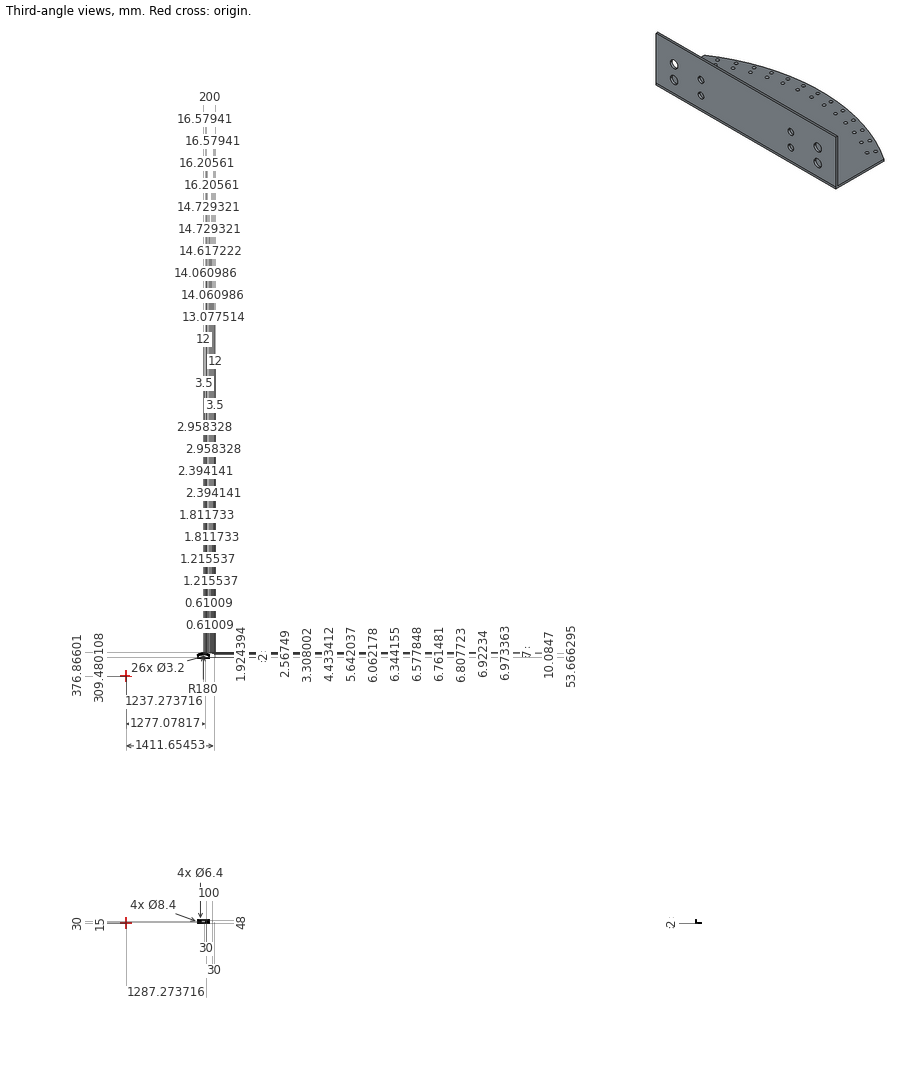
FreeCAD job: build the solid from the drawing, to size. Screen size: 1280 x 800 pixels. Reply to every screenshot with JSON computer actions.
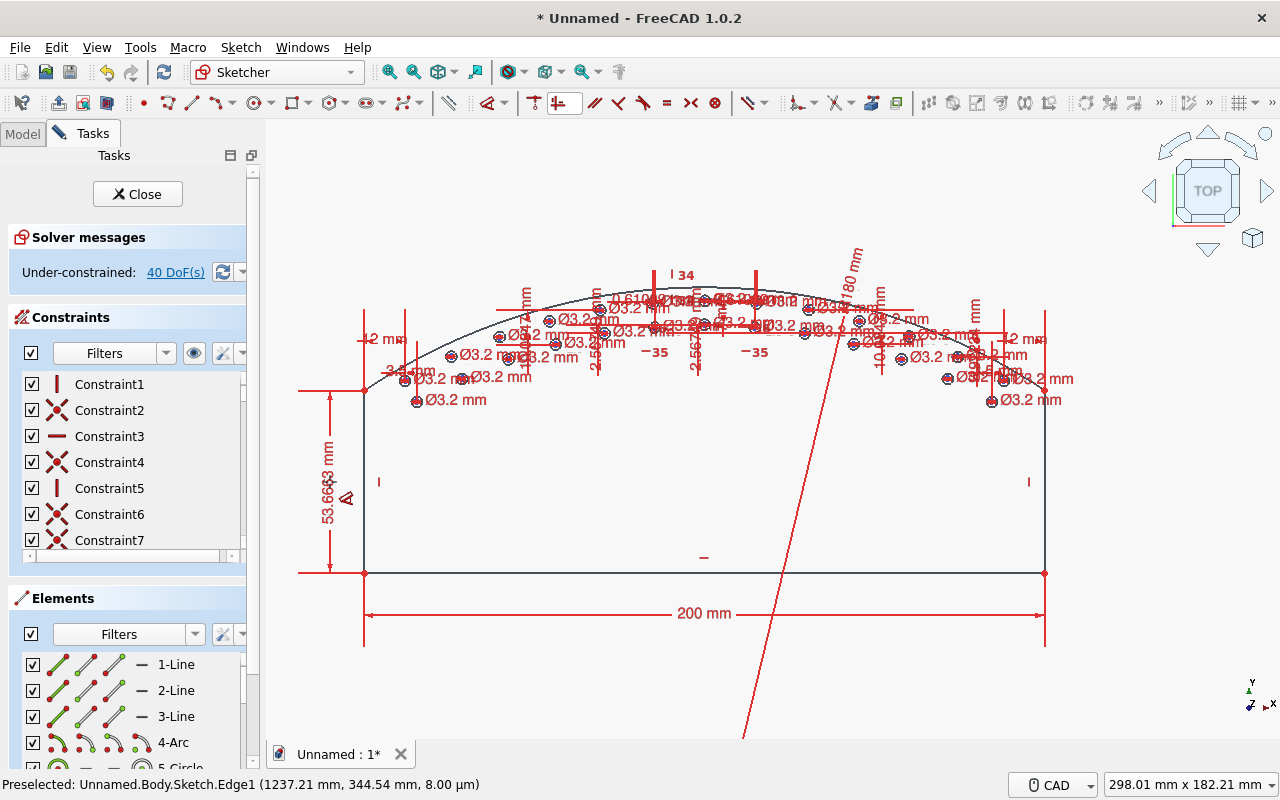
{"action": "left_click", "coordinate": [1045, 518]}
{"action": "left_click", "coordinate": [1079, 482]}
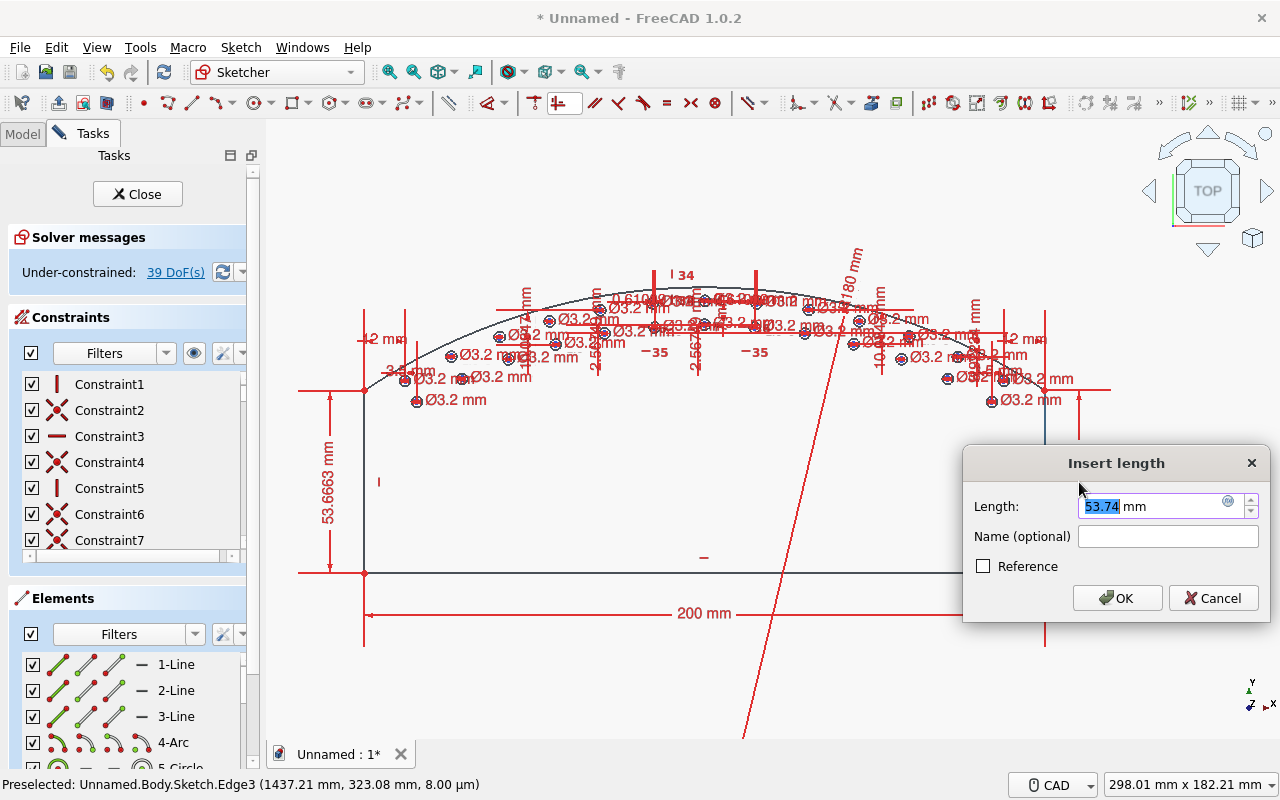
{"action": "type", "text": "53.666295"}
{"action": "key", "text": "Return"}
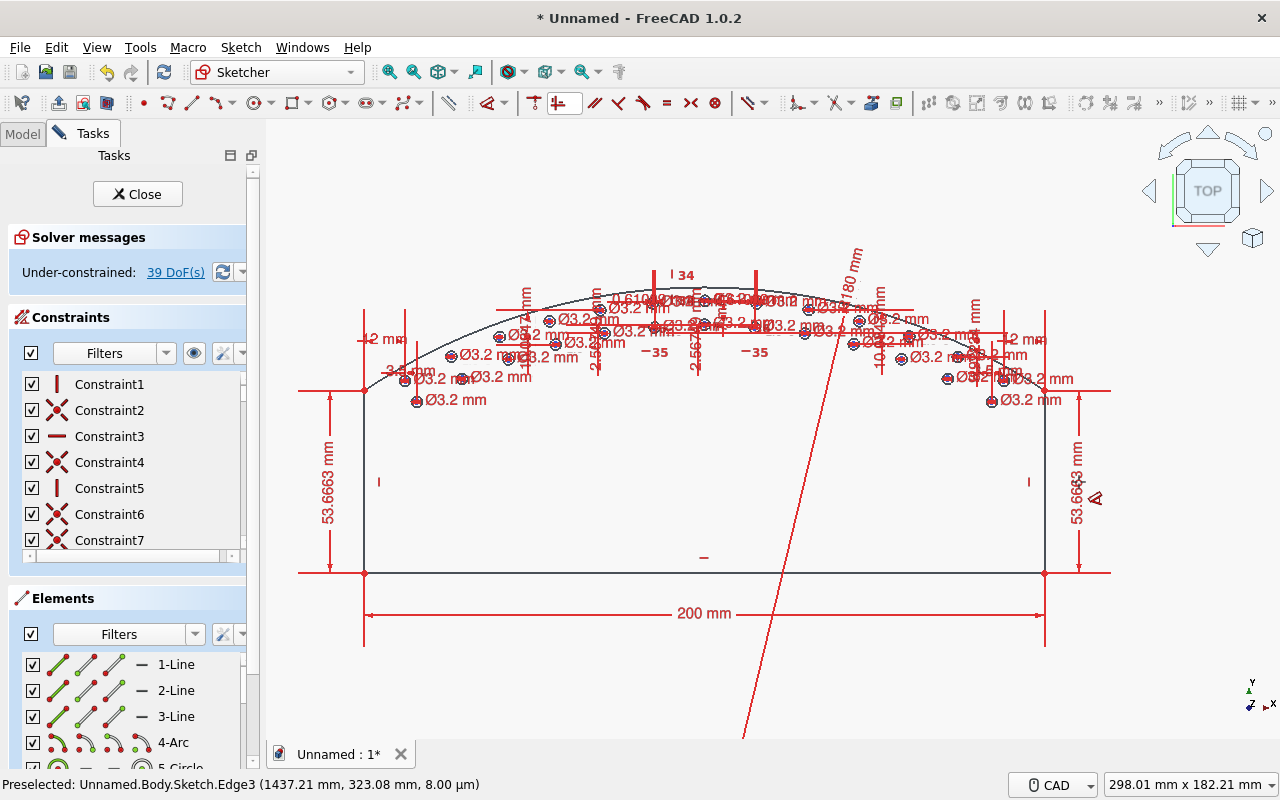
{"action": "left_click", "coordinate": [909, 337]}
{"action": "left_click", "coordinate": [943, 524]}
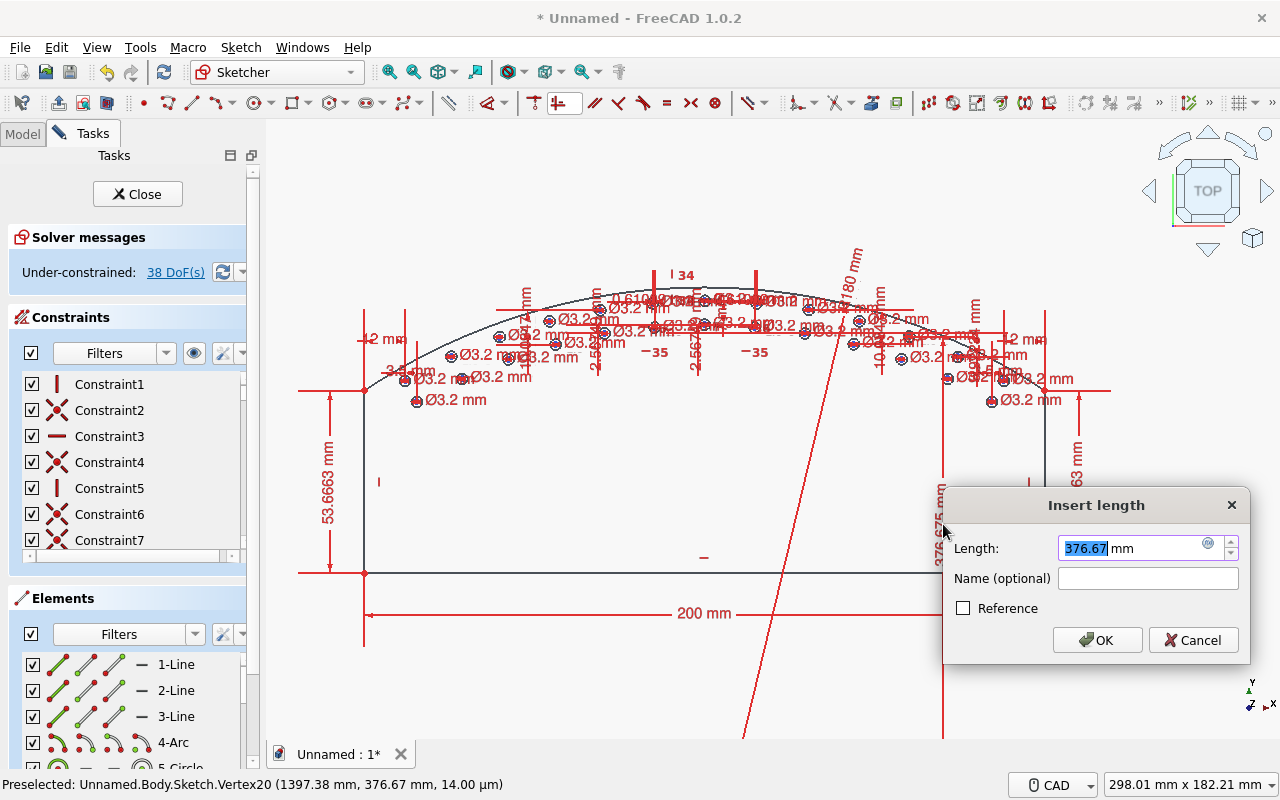
{"action": "type", "text": "376.86601"}
{"action": "key", "text": "Return"}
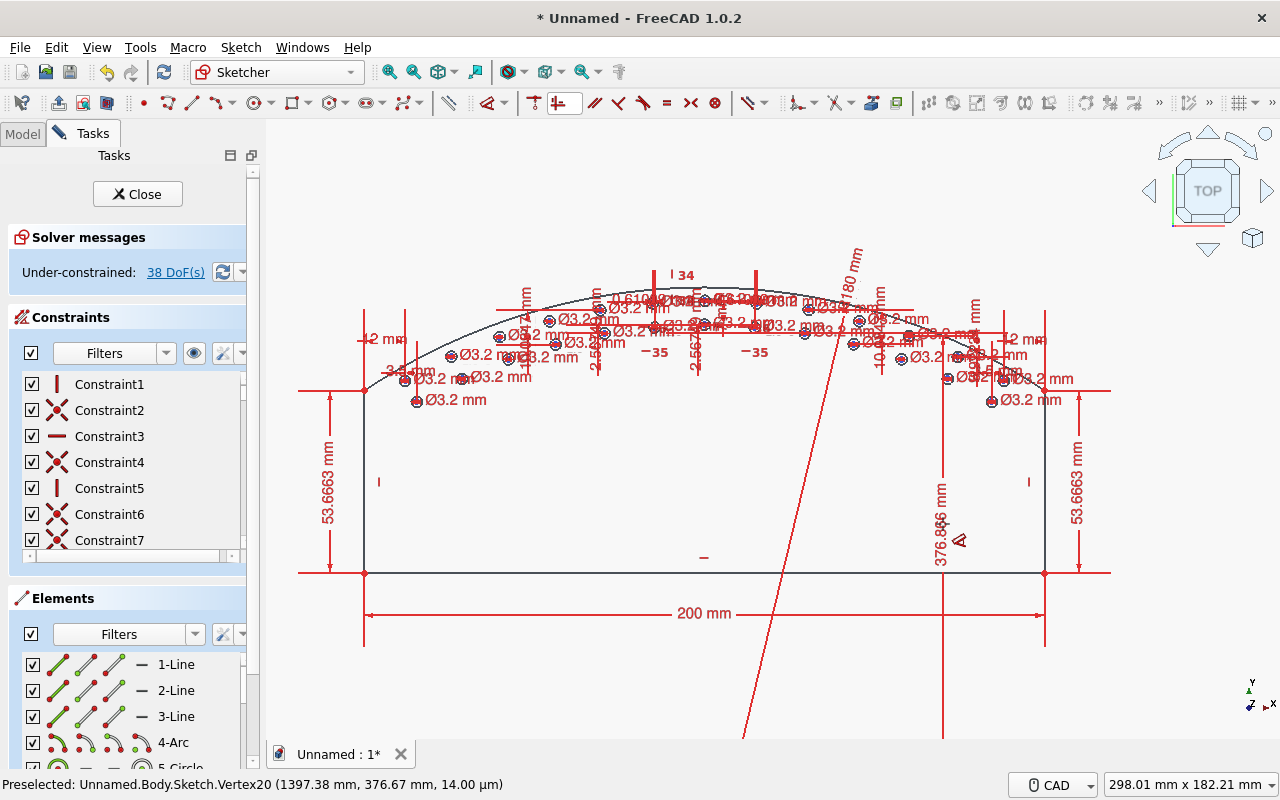
{"action": "left_click", "coordinate": [500, 337]}
{"action": "left_click", "coordinate": [534, 524]}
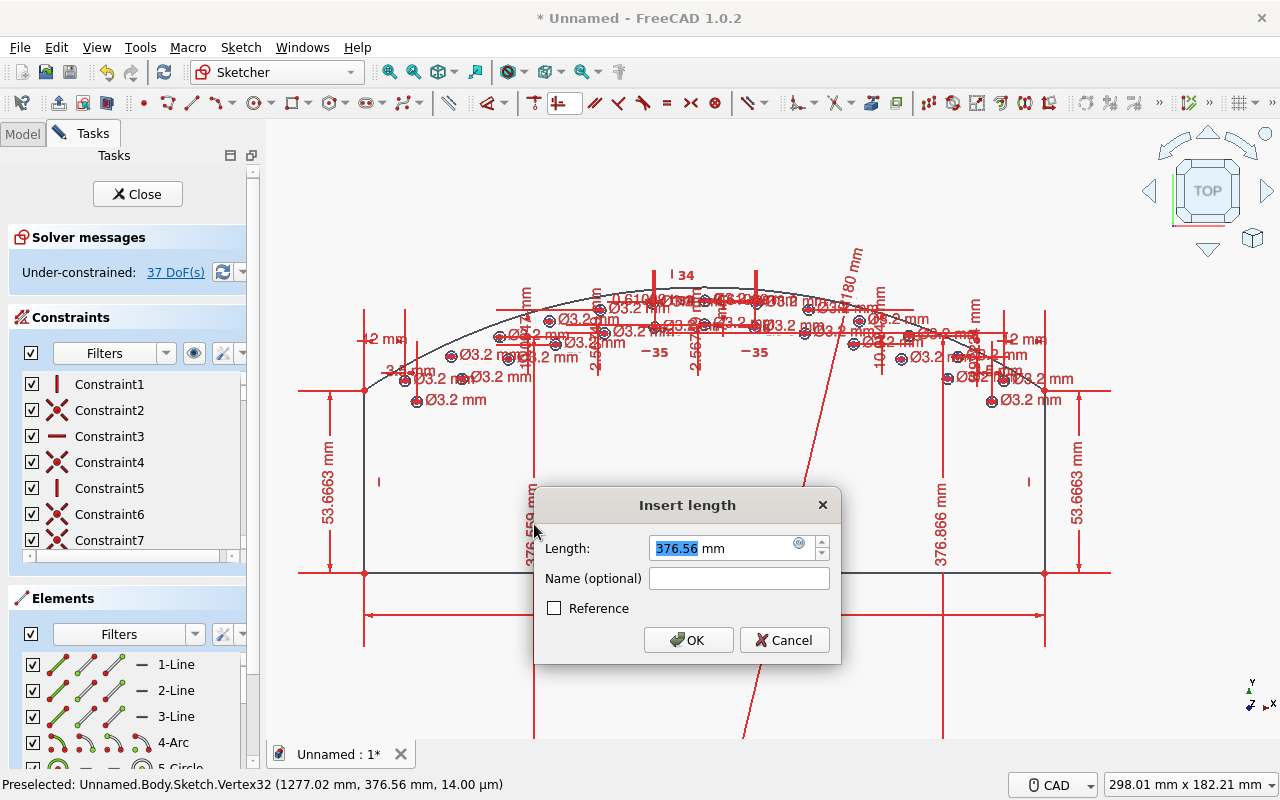
{"action": "type", "text": "376.86601"}
{"action": "key", "text": "Return"}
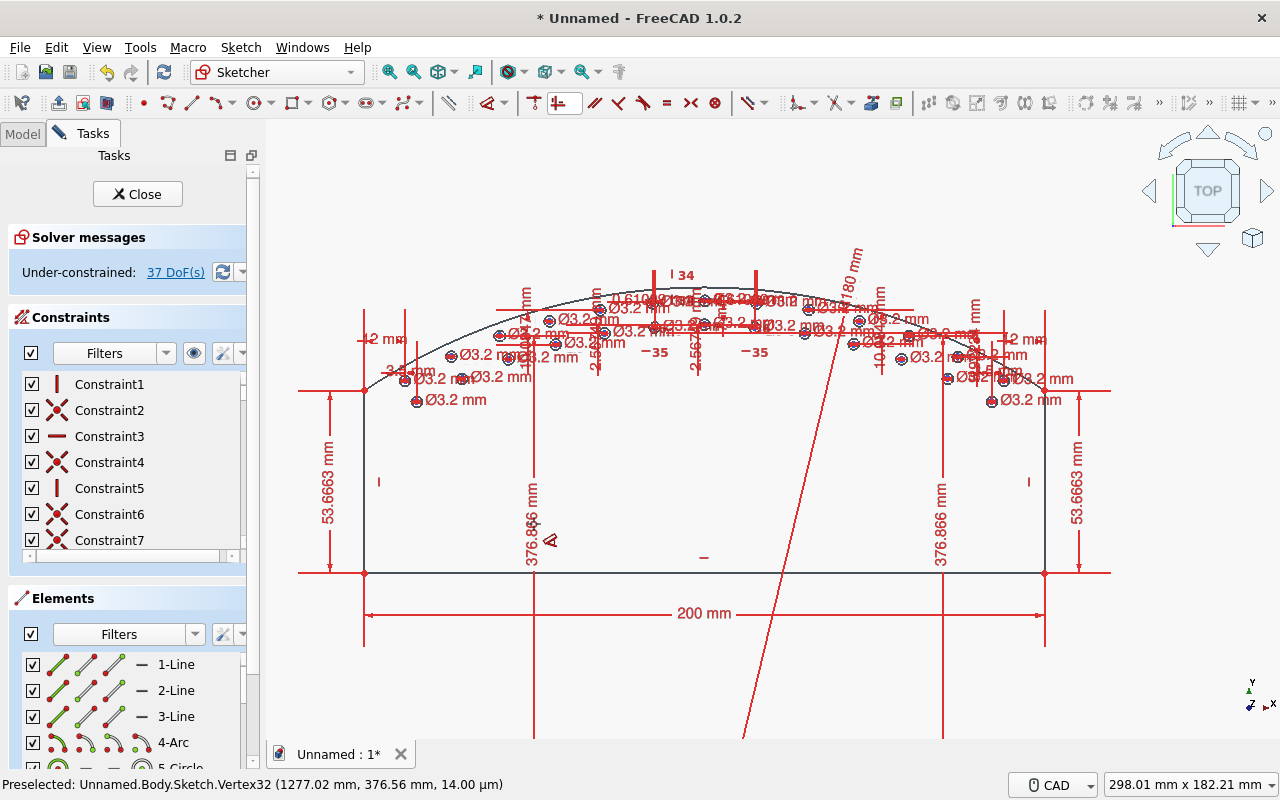
{"action": "scroll", "coordinate": [1045, 391], "scroll_direction": "up", "scroll_amount": 7}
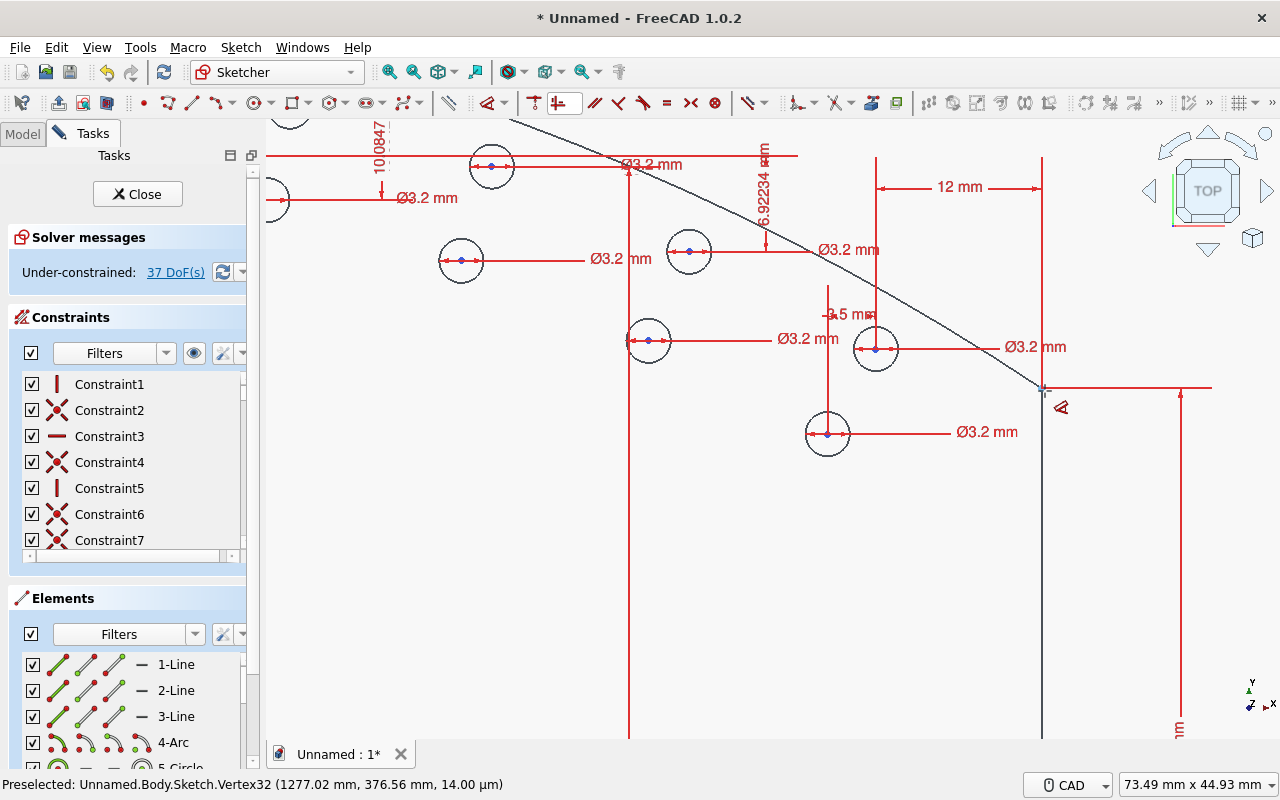
{"action": "left_click", "coordinate": [1042, 388]}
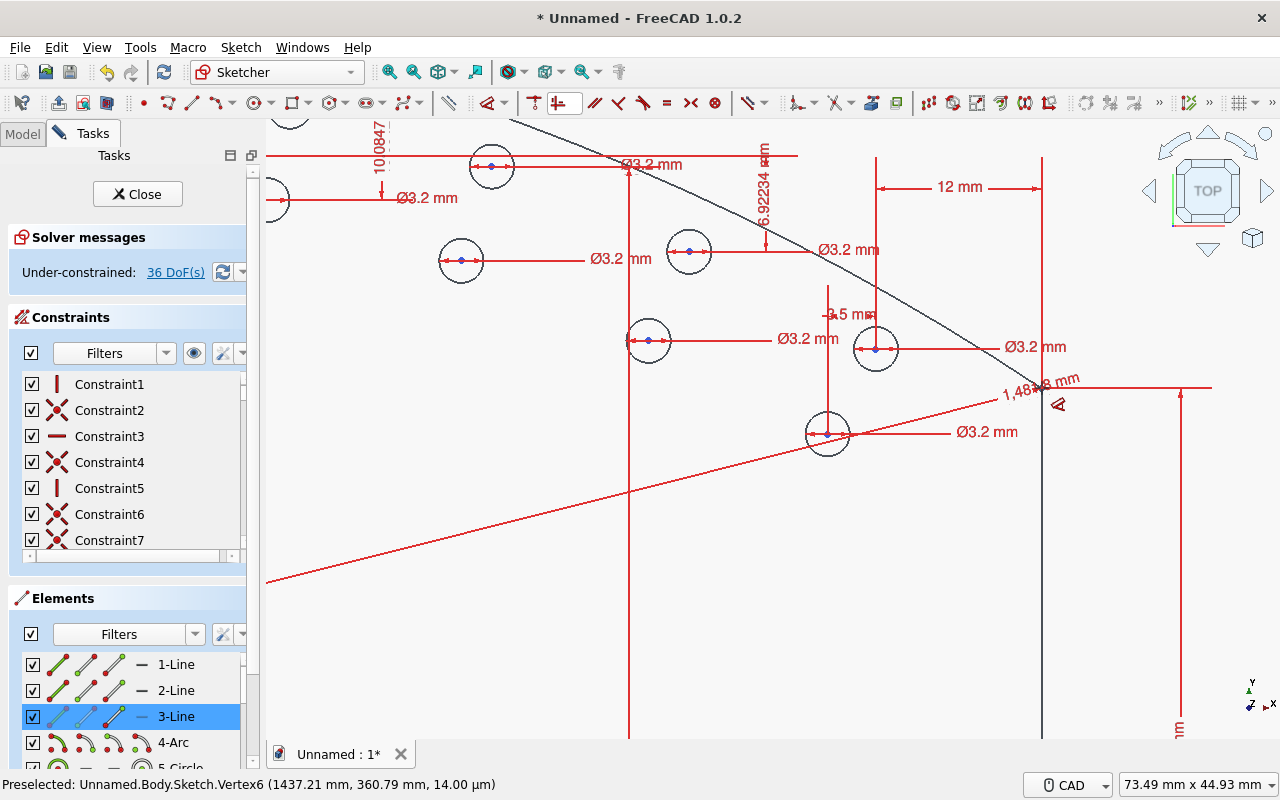
{"action": "left_click", "coordinate": [828, 434]}
{"action": "left_click", "coordinate": [1076, 411]}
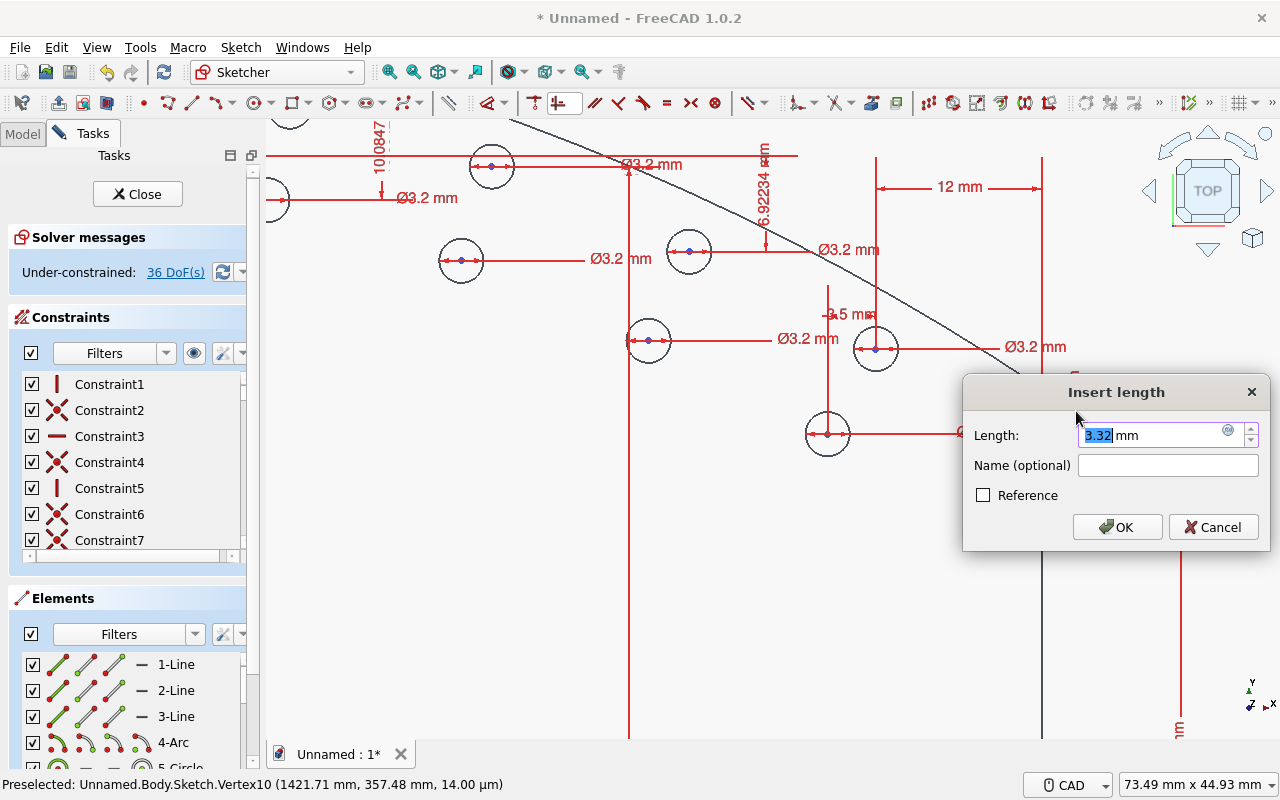
{"action": "type", "text": "3.308002"}
{"action": "key", "text": "Return"}